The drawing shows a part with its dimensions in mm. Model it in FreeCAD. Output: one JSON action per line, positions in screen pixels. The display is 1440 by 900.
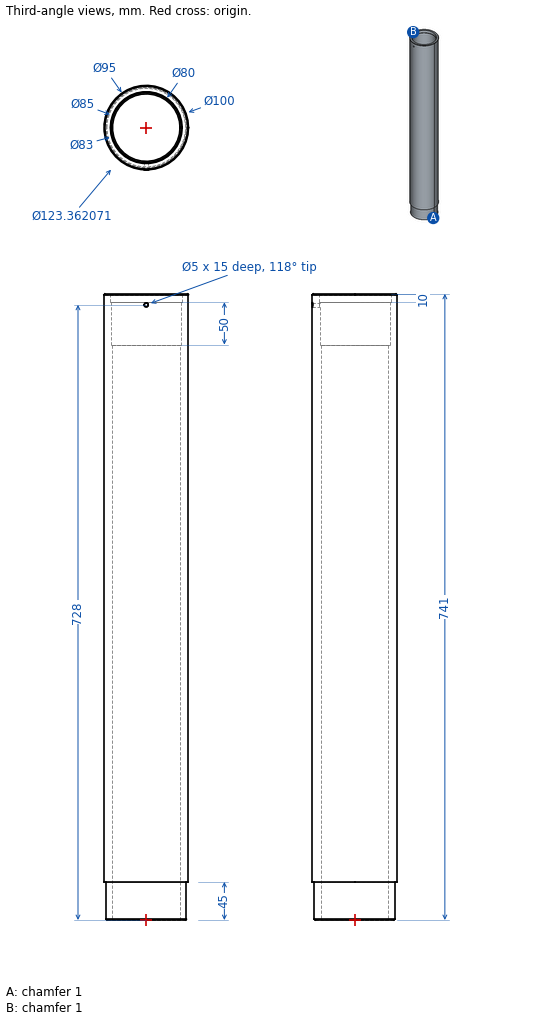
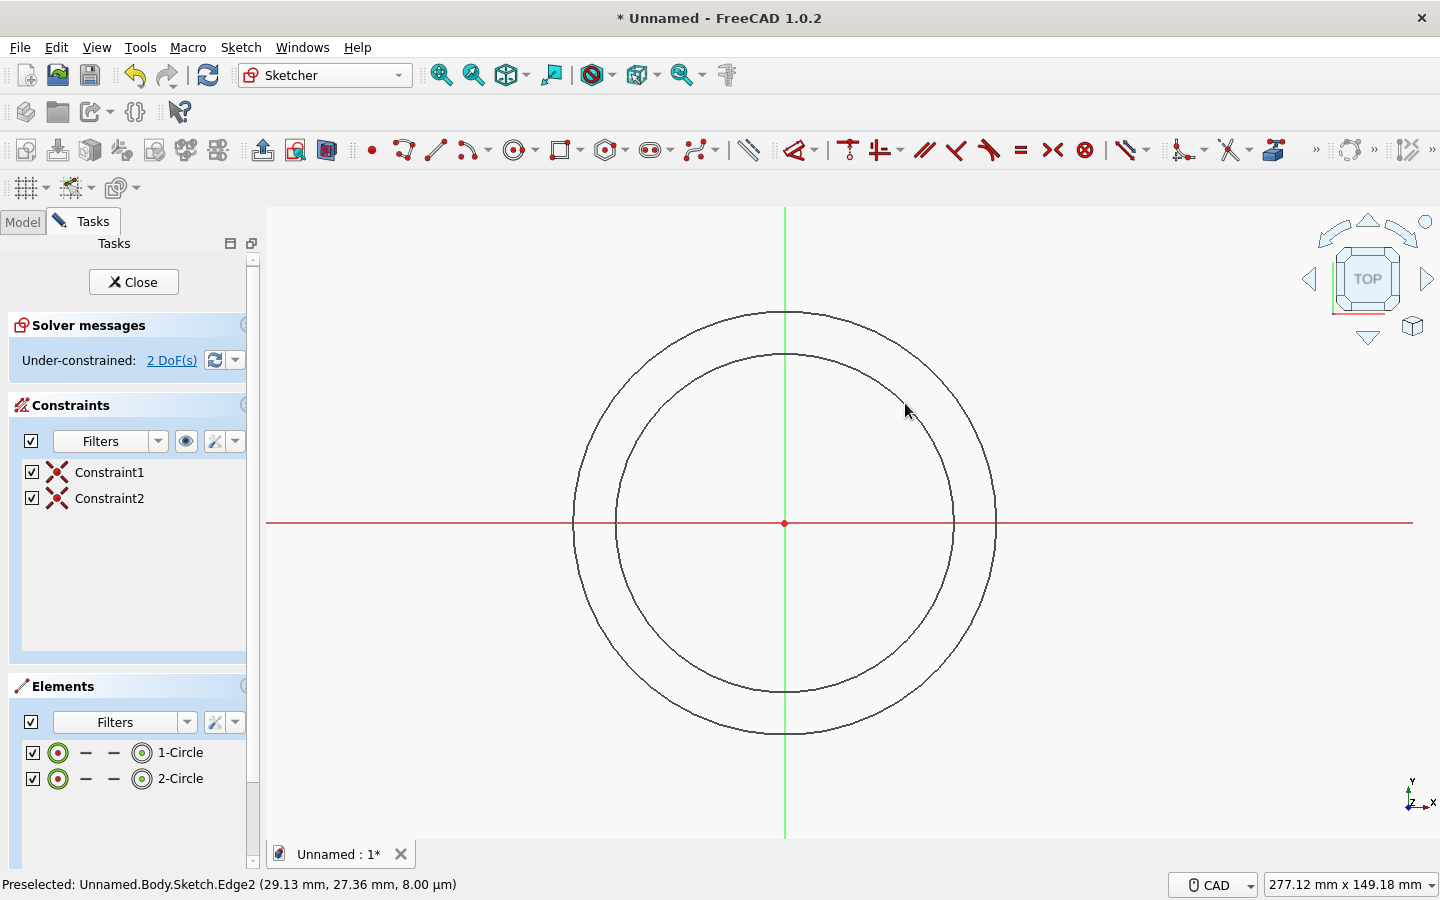
{"action": "left_click", "coordinate": [934, 373]}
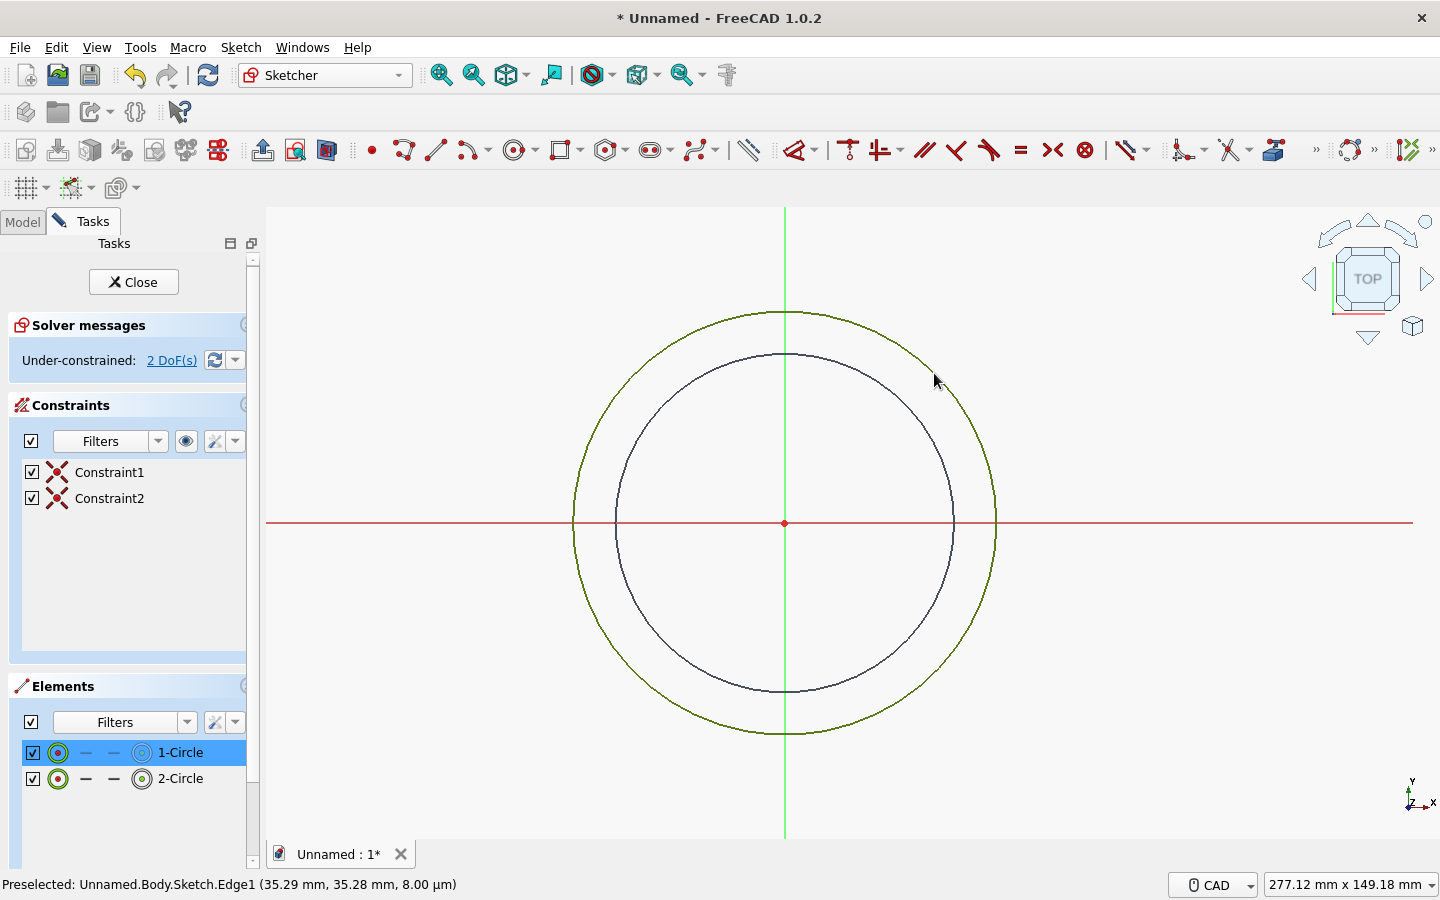
{"action": "key", "text": "k o"}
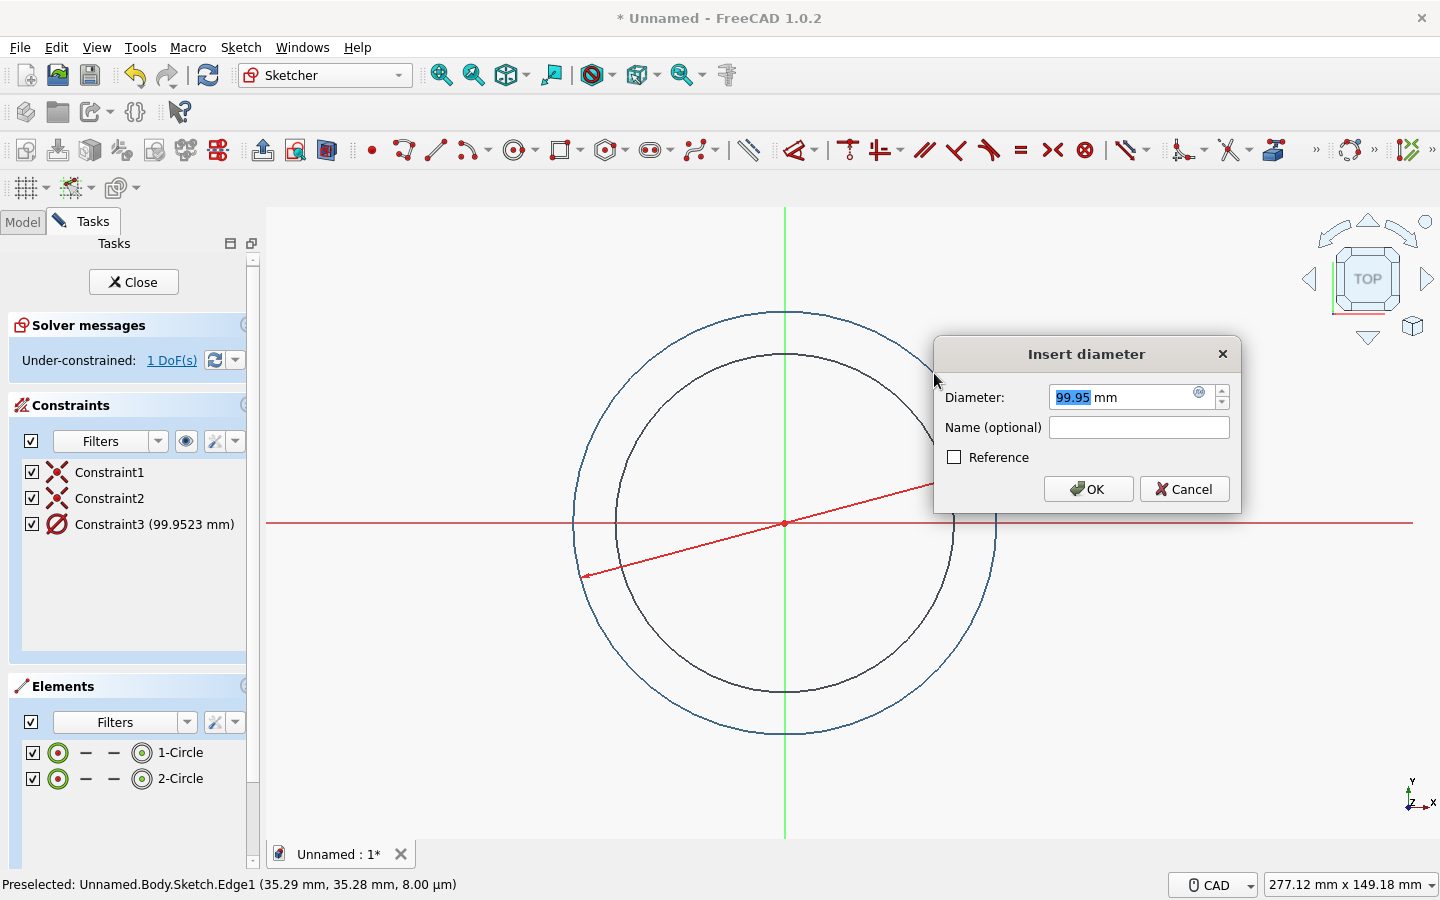
{"action": "type", "text": "100"}
{"action": "key", "text": "Return"}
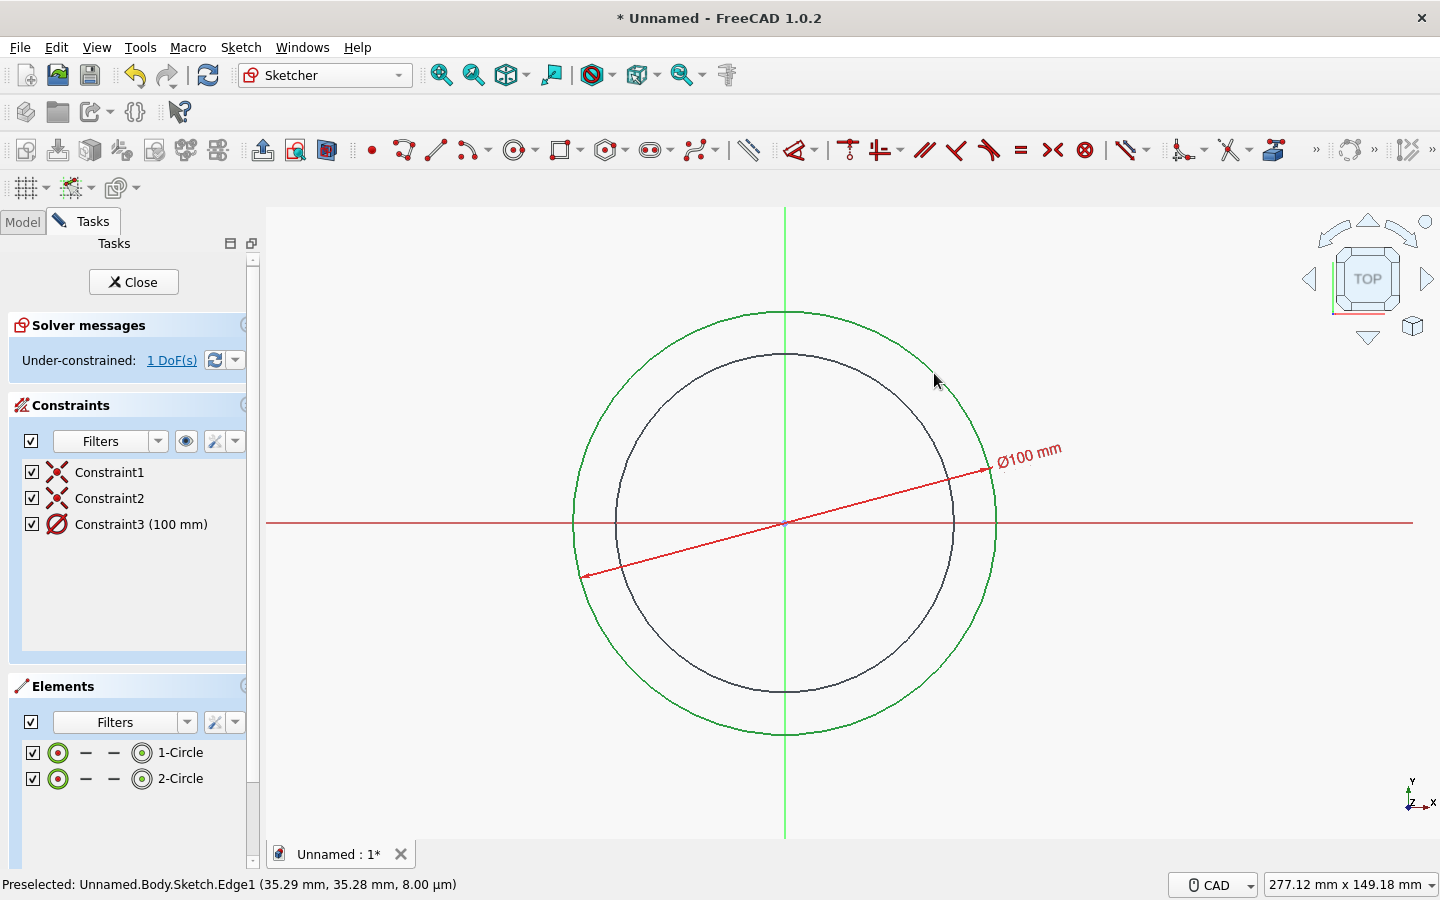
{"action": "left_click", "coordinate": [904, 403]}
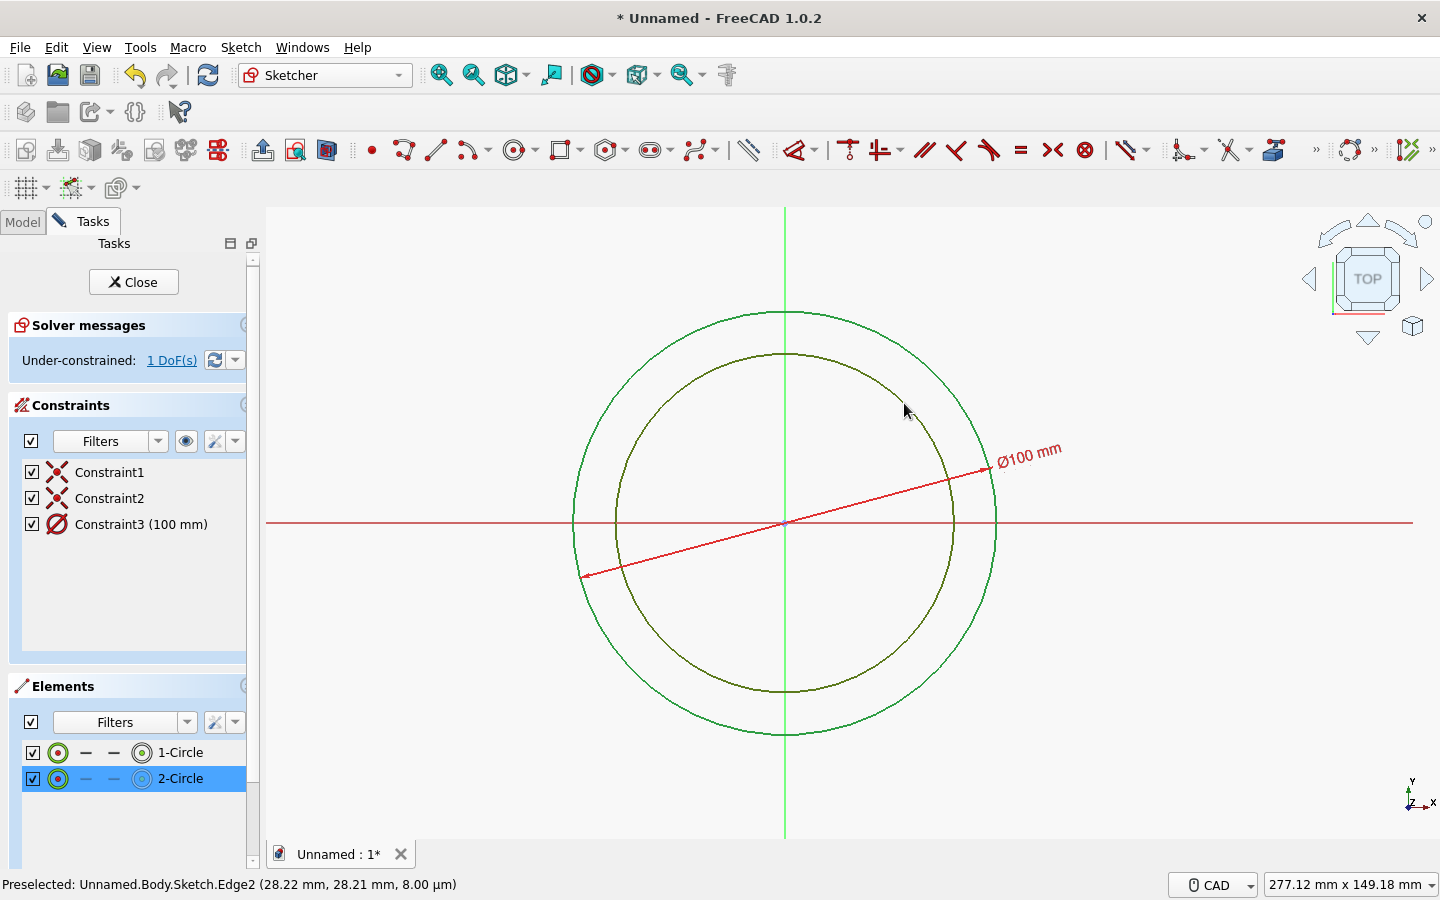
{"action": "left_click", "coordinate": [816, 150]}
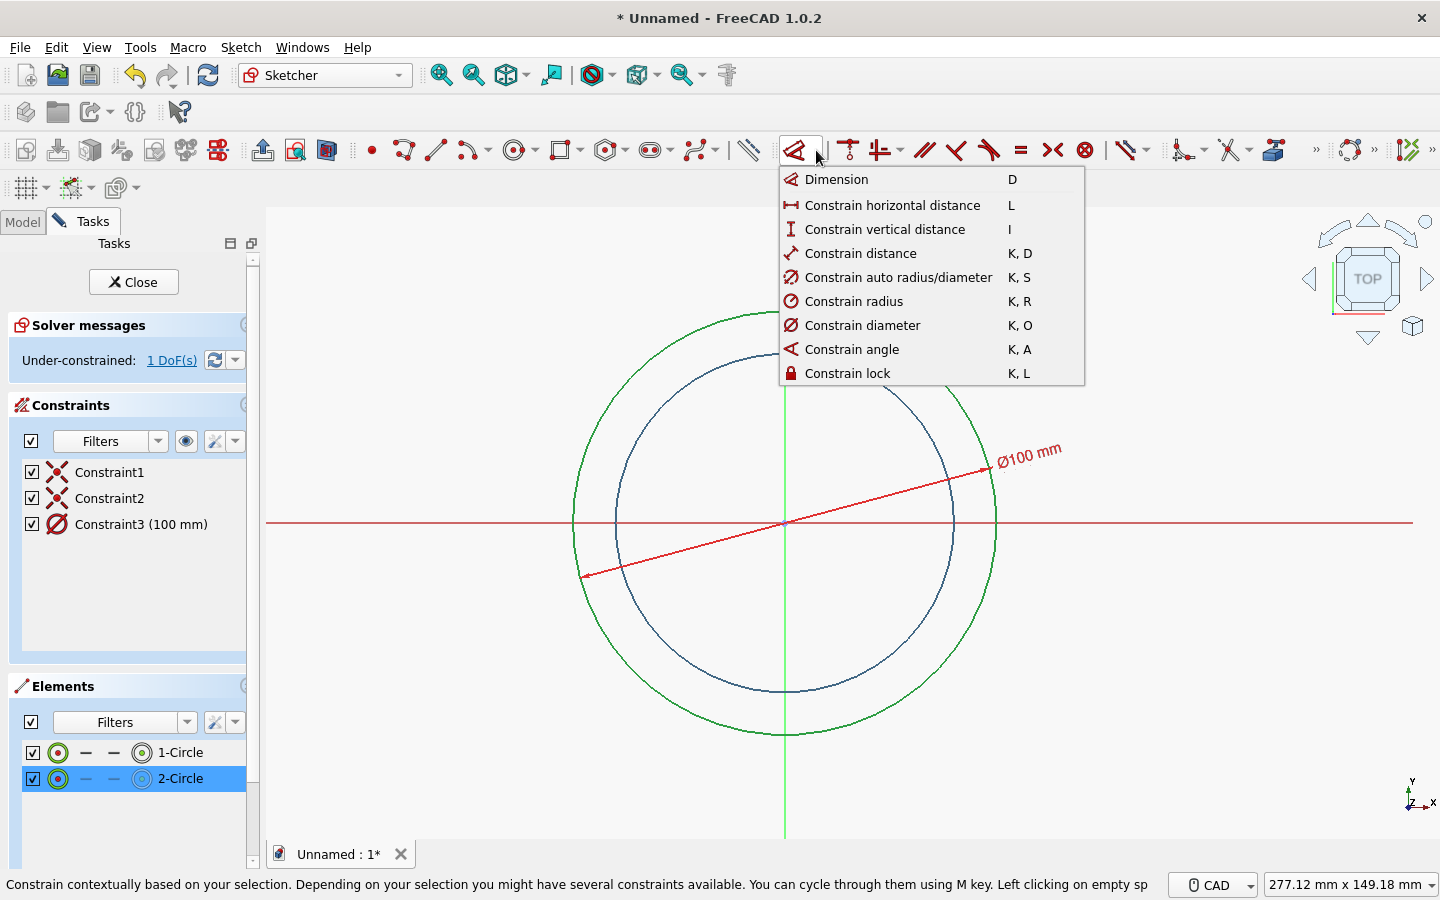
{"action": "left_click", "coordinate": [932, 325]}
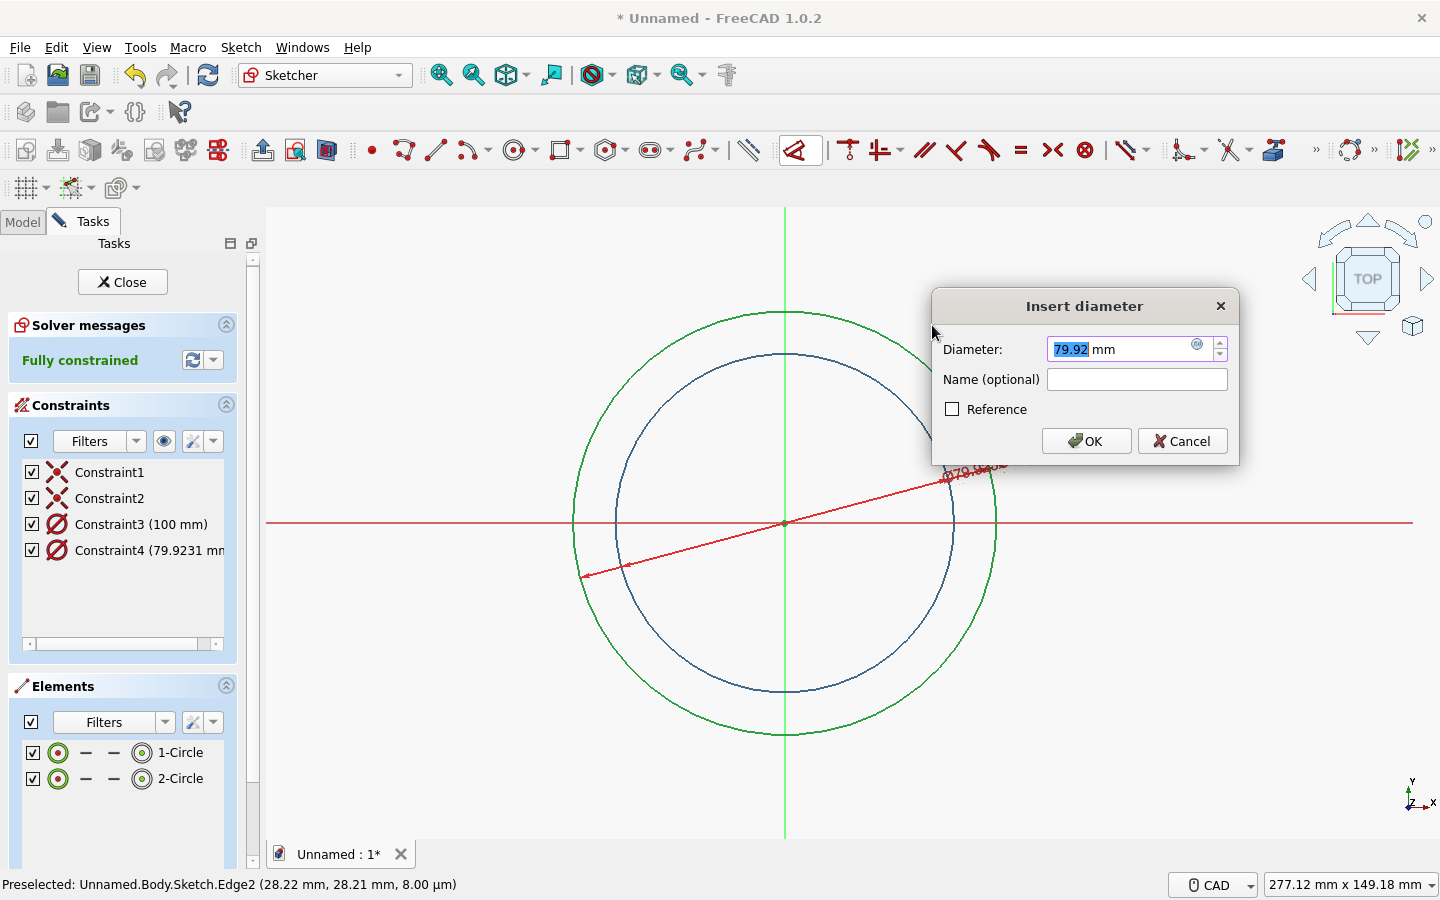
{"action": "type", "text": "80"}
{"action": "key", "text": "Return"}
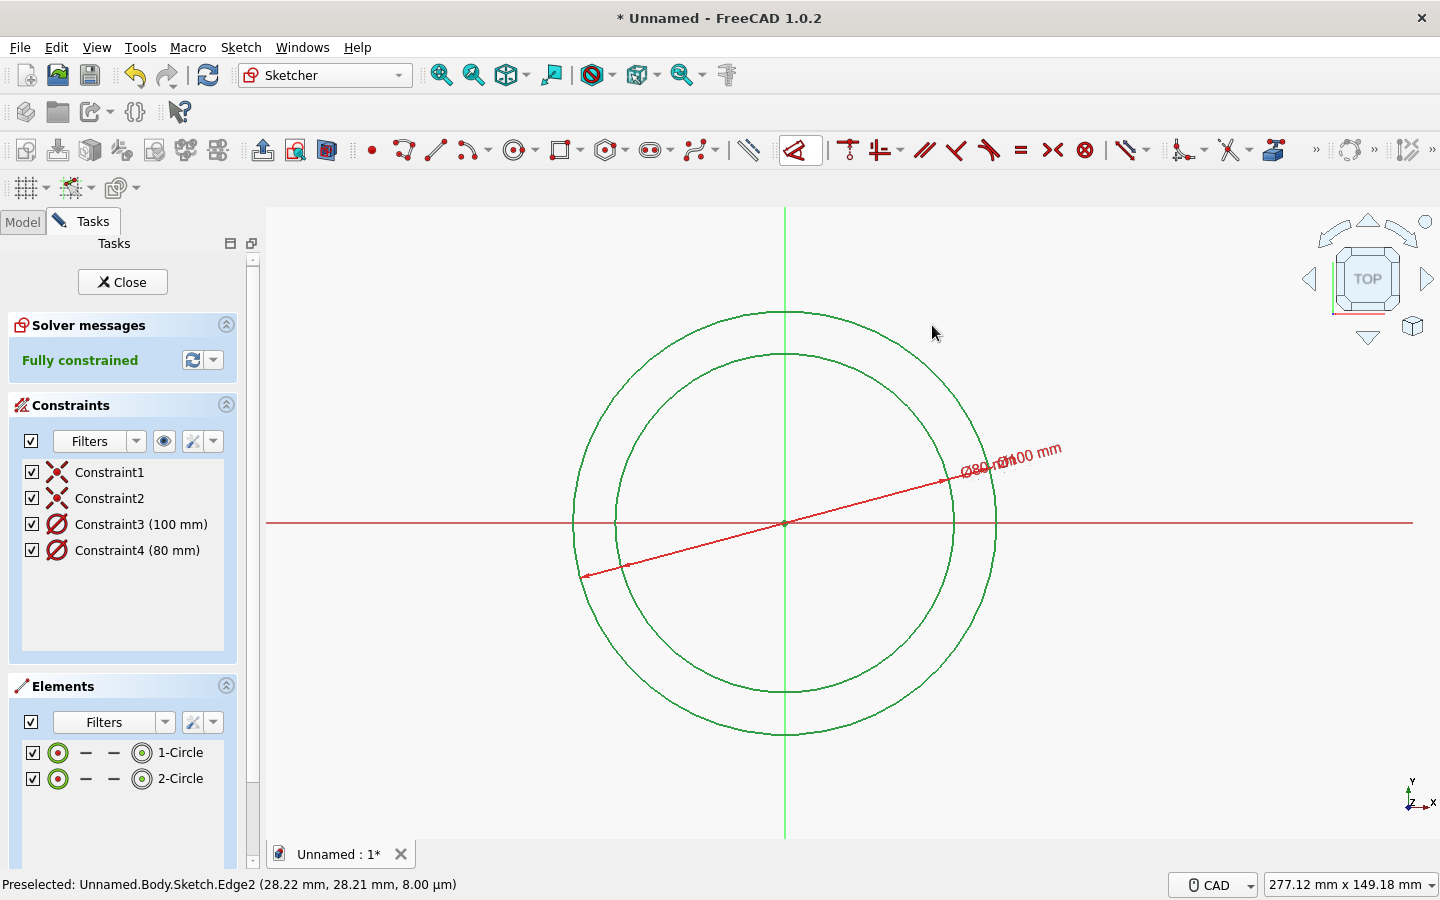
{"action": "left_click", "coordinate": [123, 282]}